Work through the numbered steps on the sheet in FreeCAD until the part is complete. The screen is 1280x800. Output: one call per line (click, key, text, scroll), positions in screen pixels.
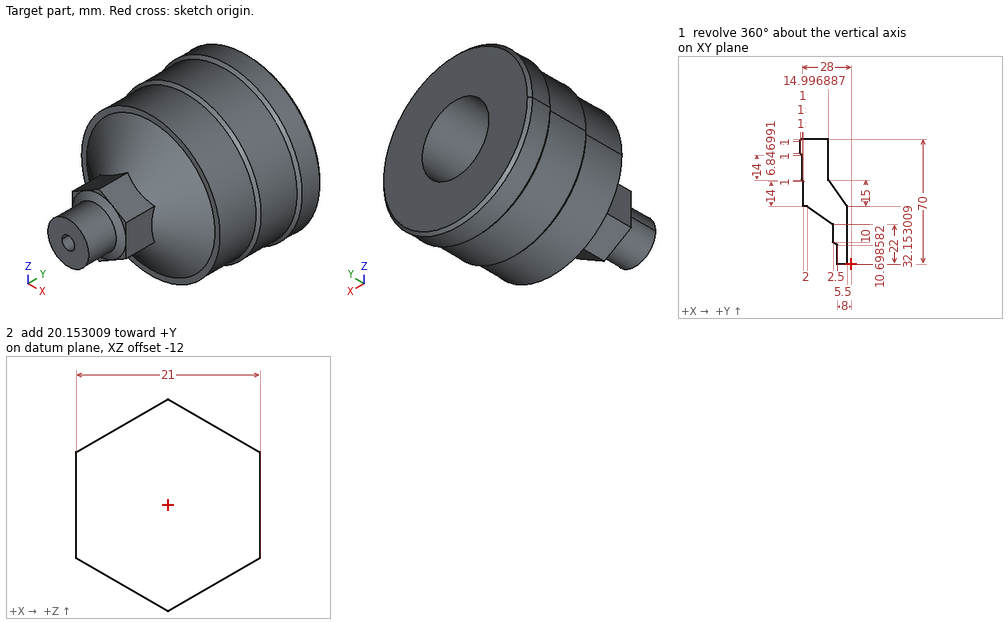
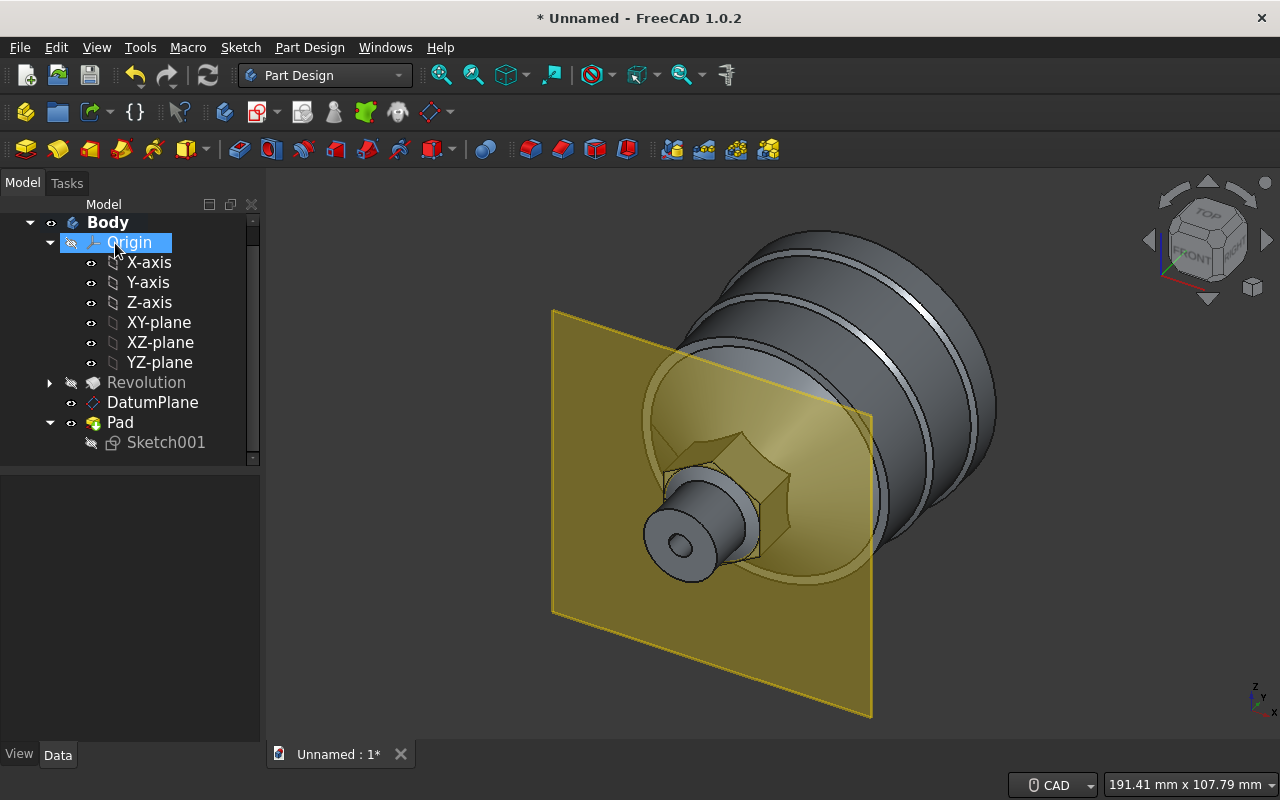
click(116, 403)
key(space)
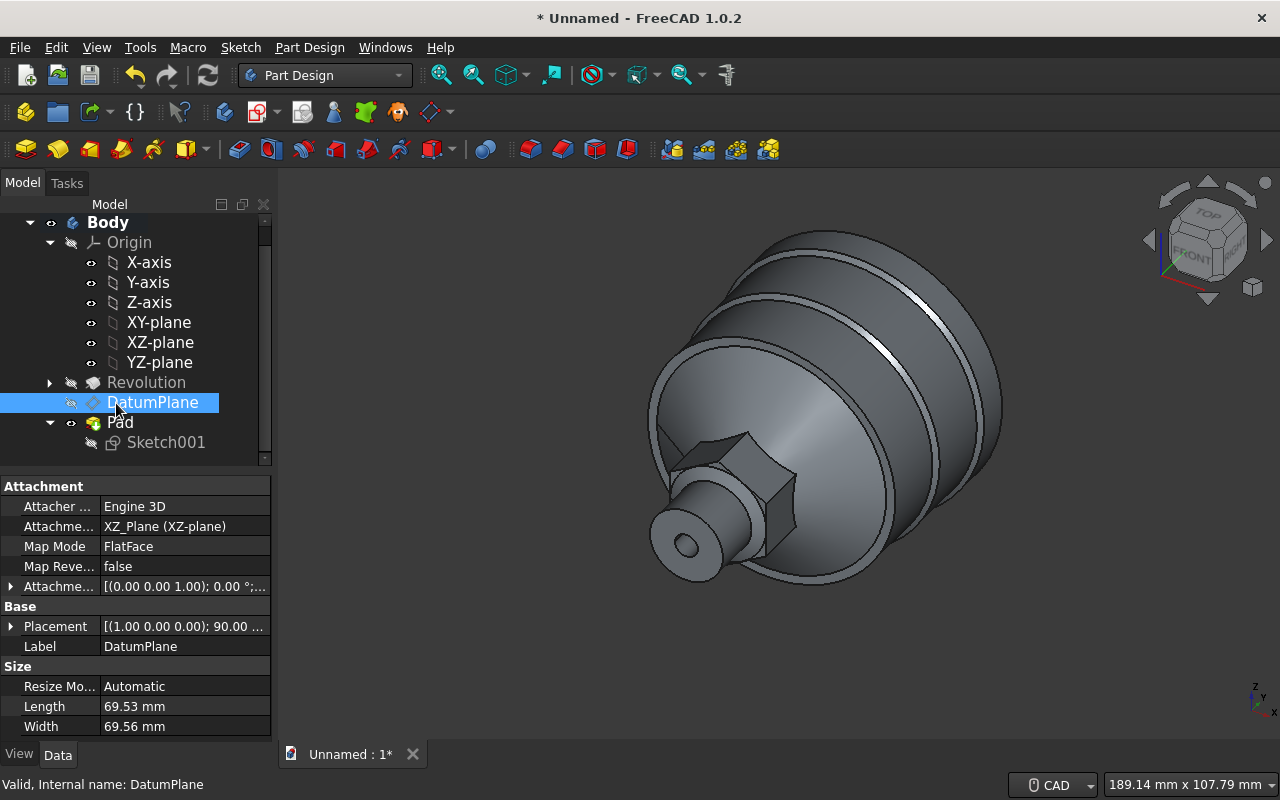
key(0)